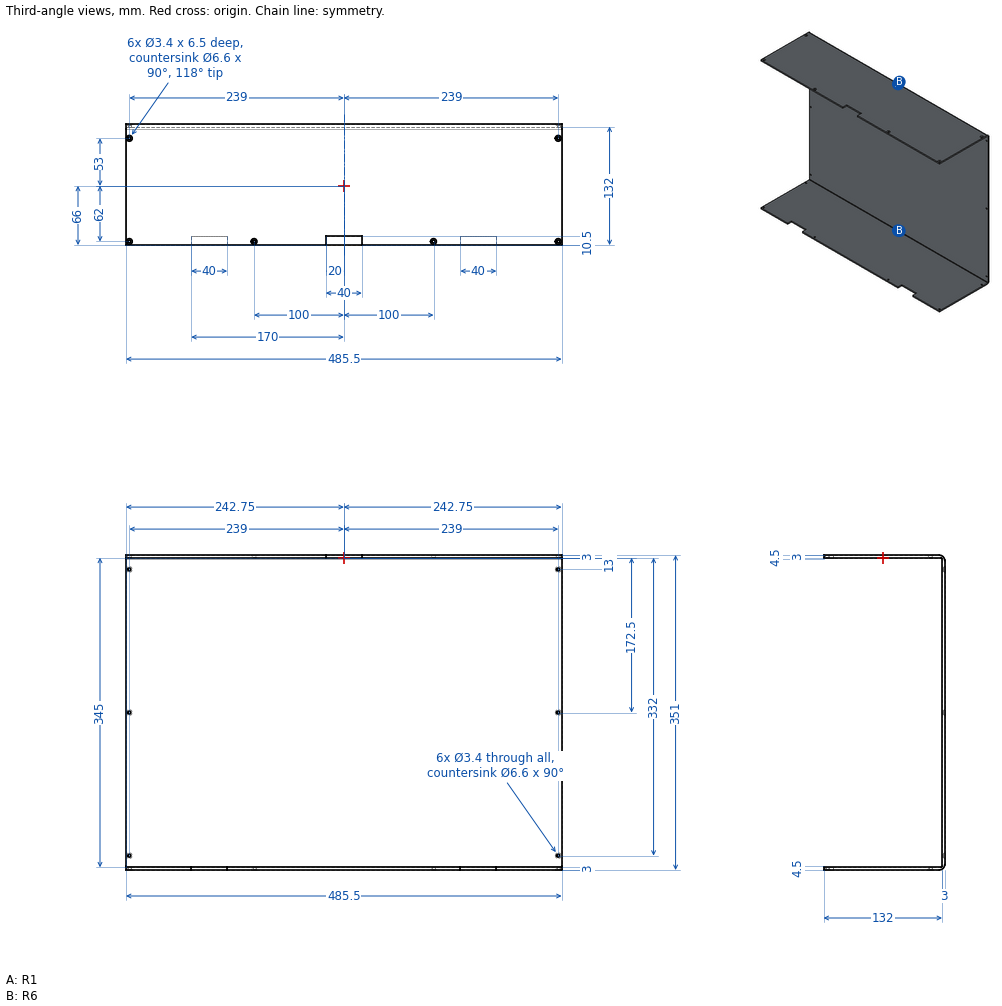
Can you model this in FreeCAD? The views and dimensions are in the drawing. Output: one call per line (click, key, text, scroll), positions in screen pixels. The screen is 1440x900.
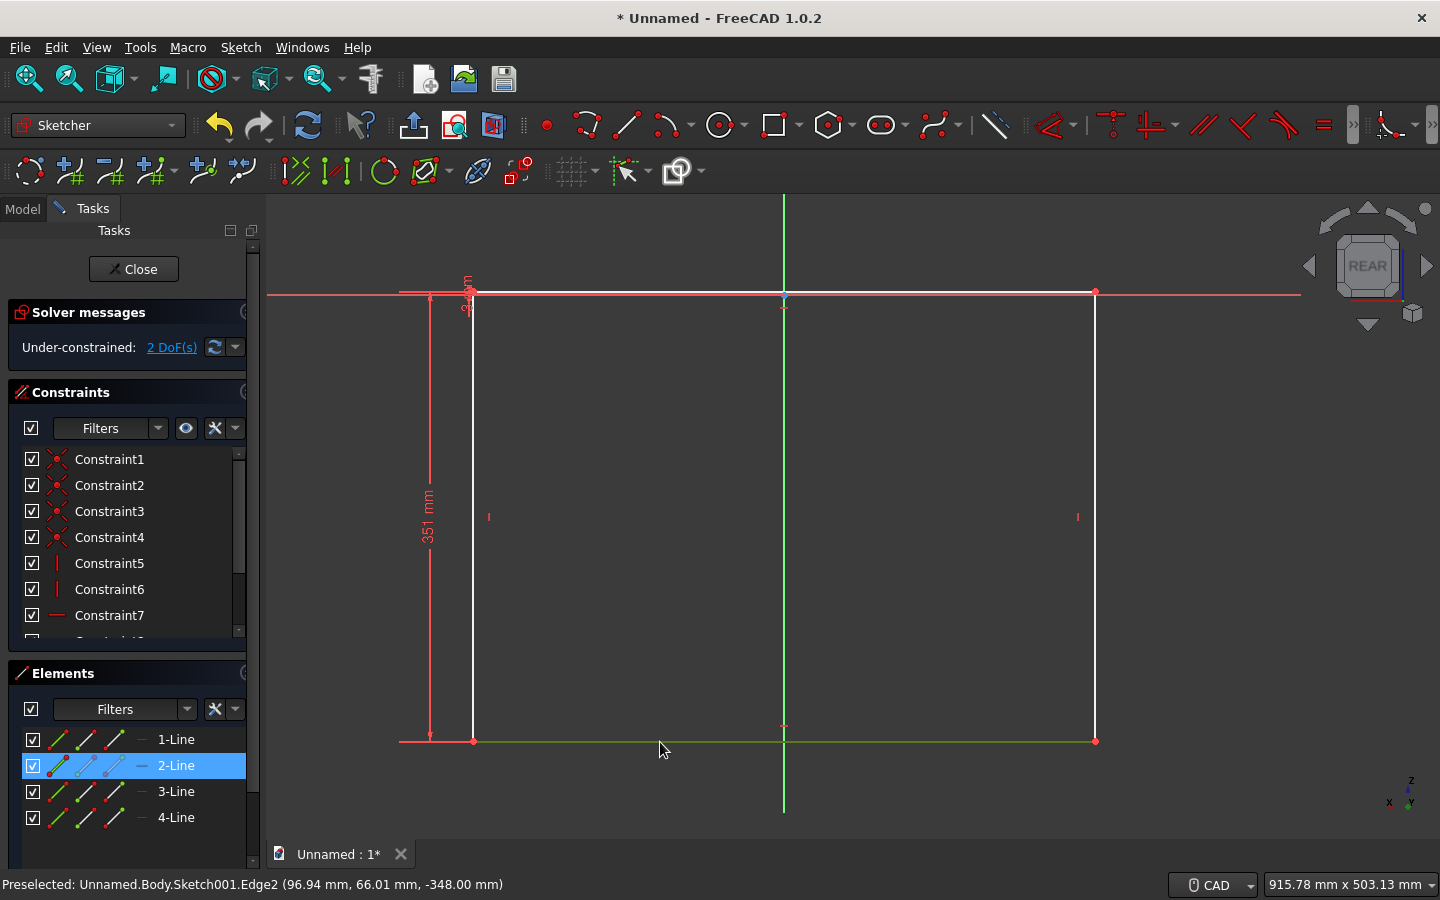
click(1076, 126)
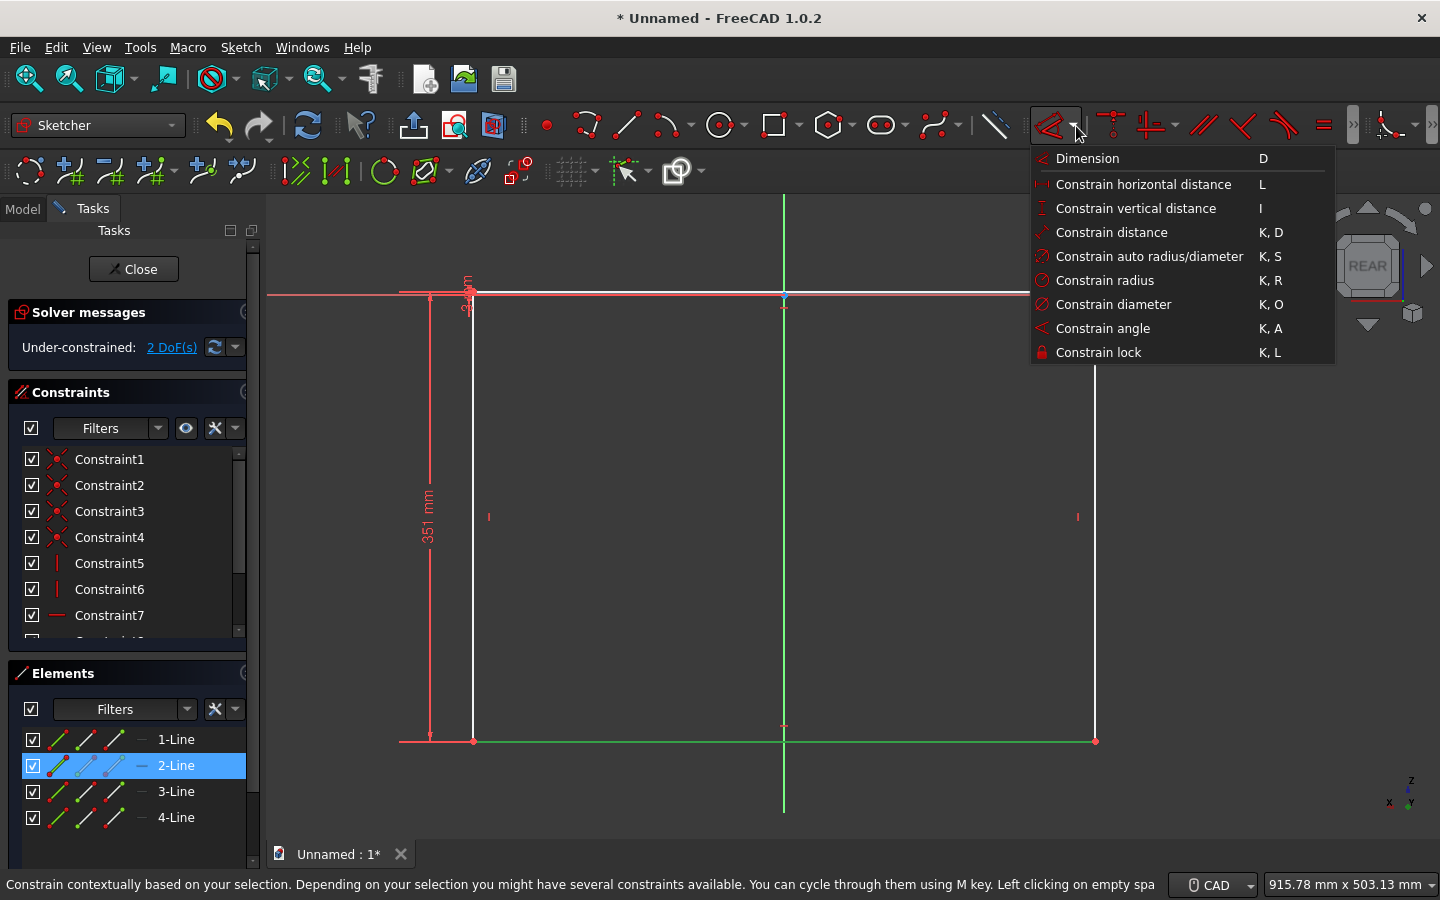
click(1183, 184)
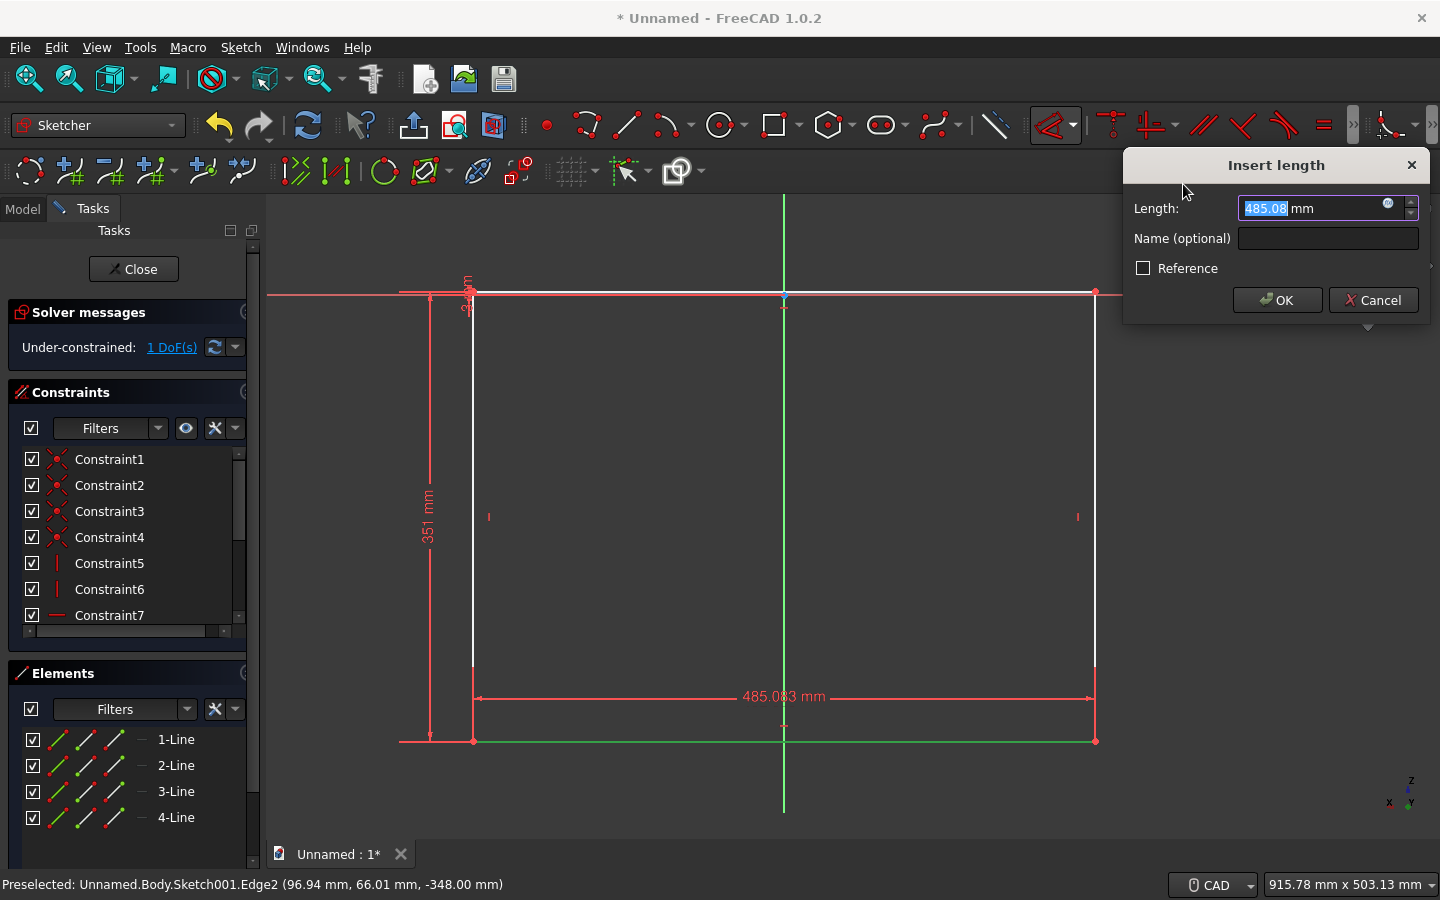
text(485.5)
key(Return)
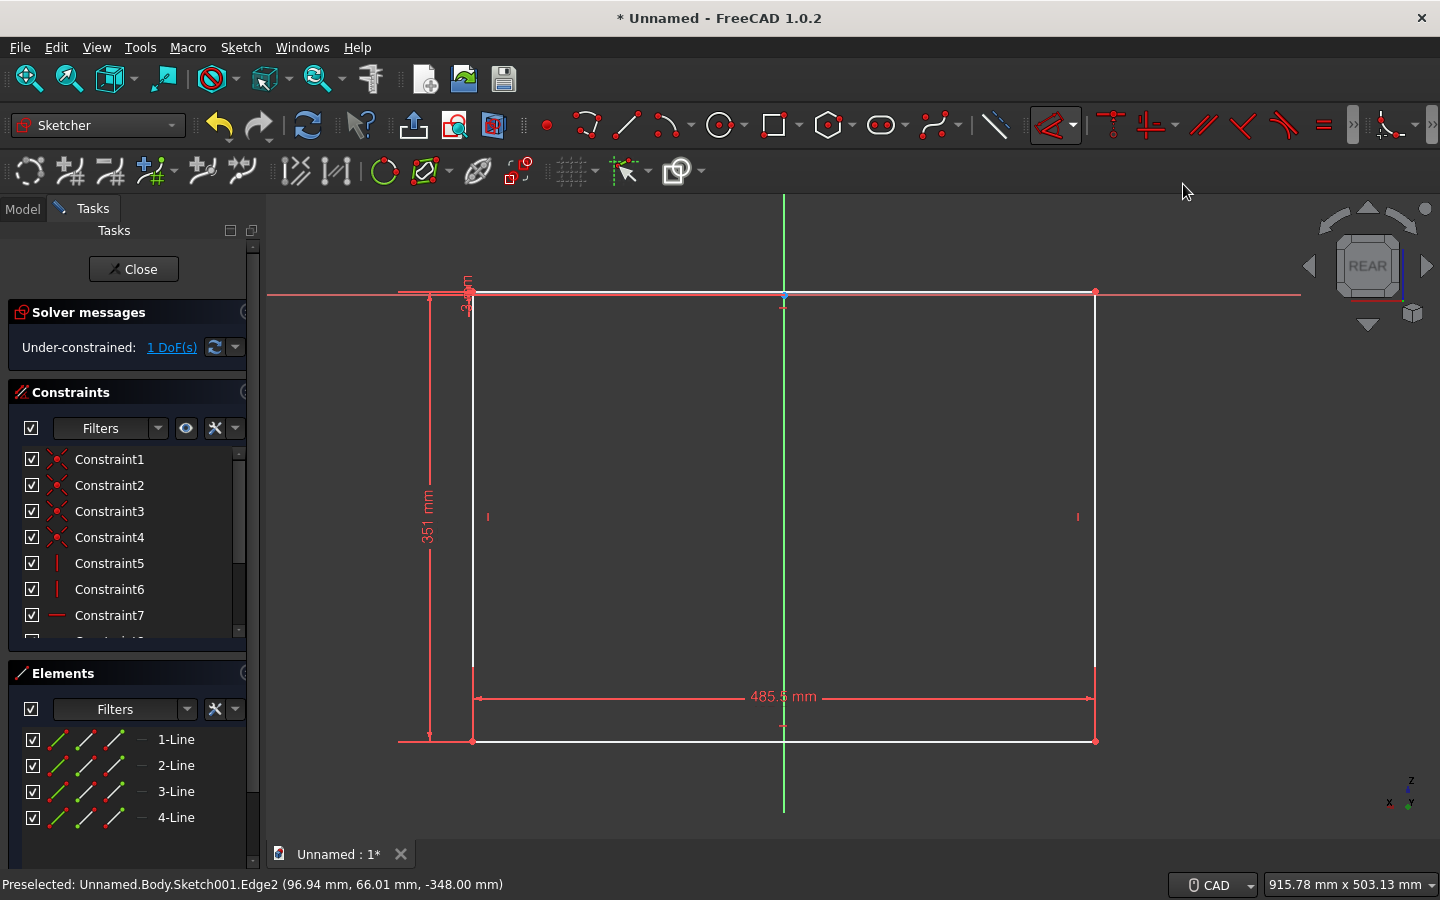
click(473, 292)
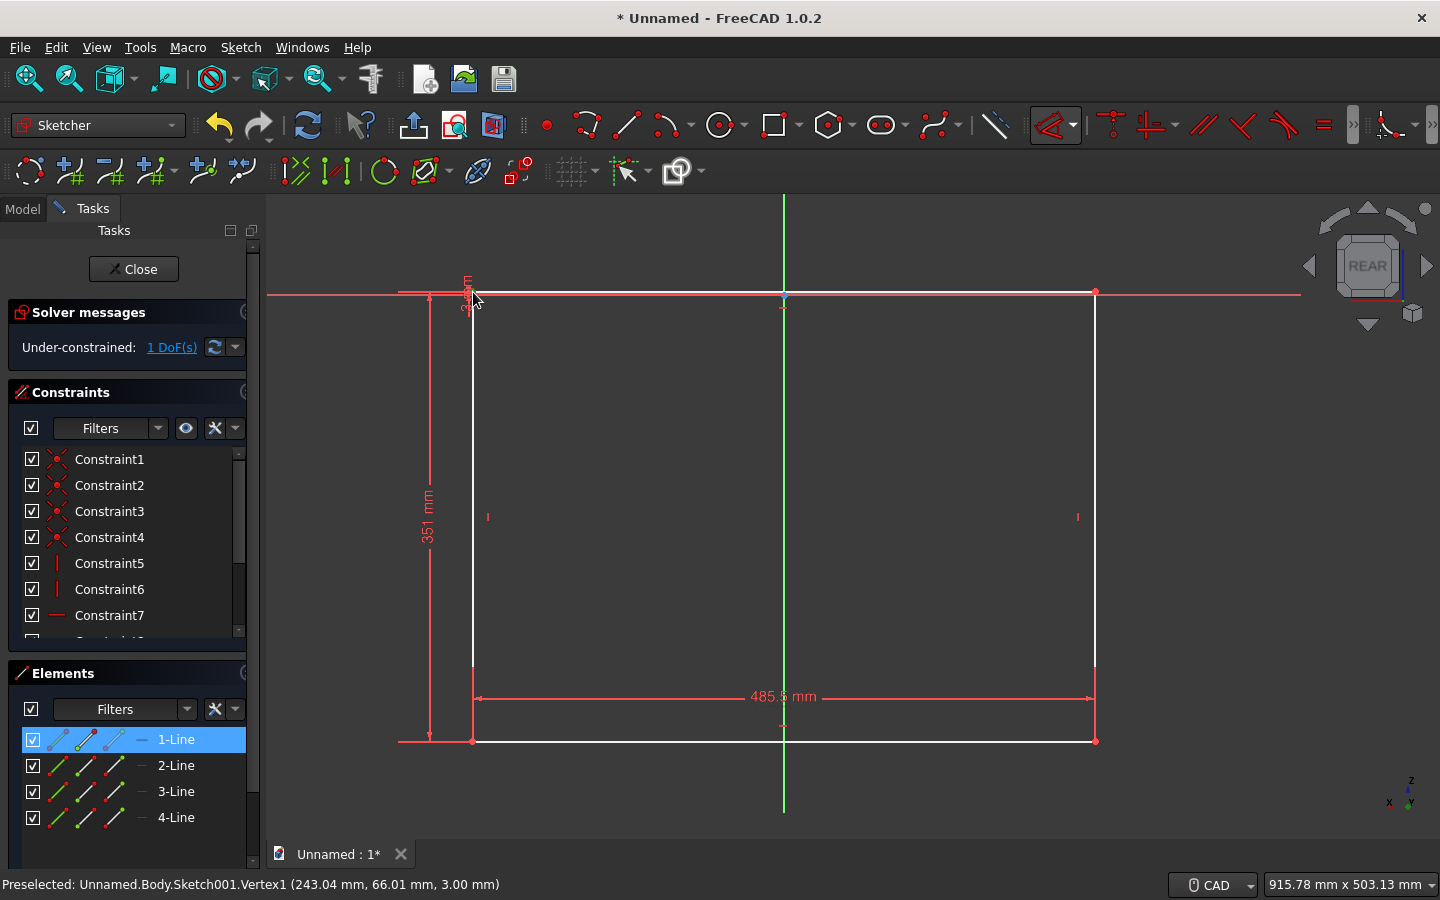
click(1076, 126)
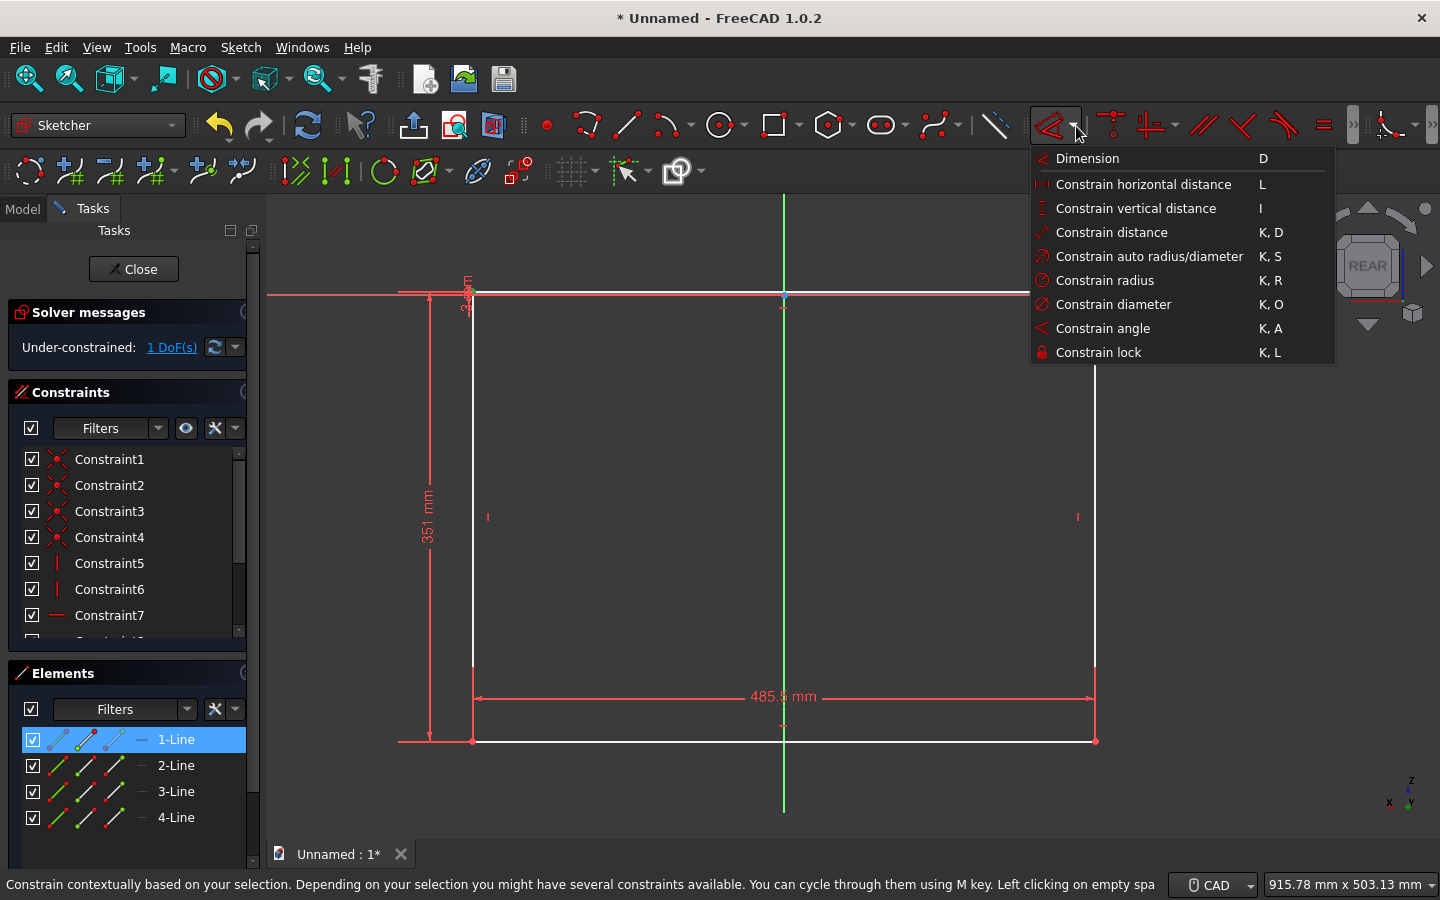
click(1183, 184)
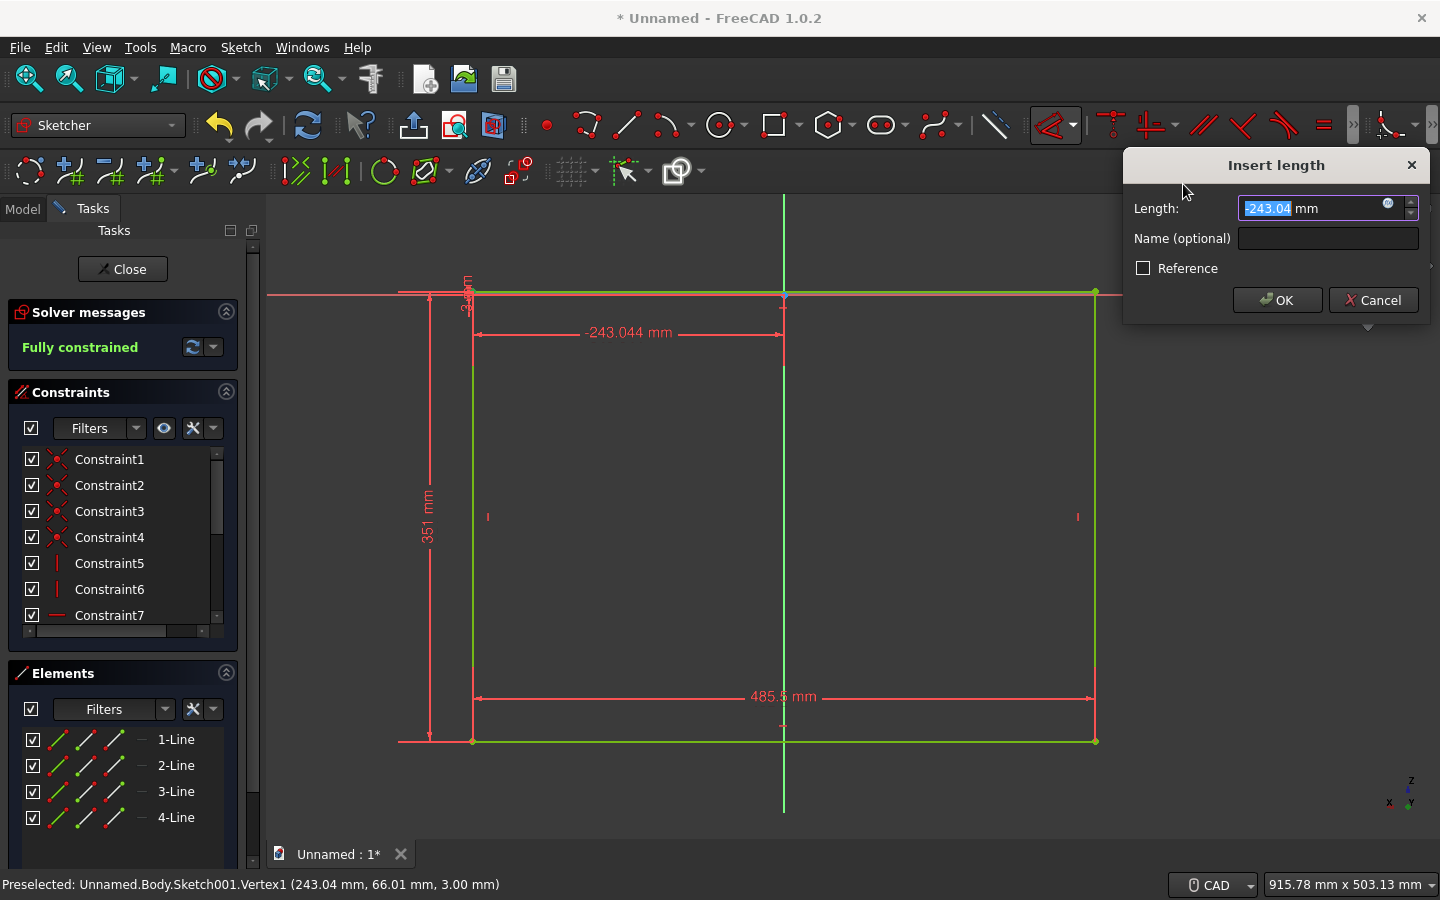
text(-242.75)
key(Return)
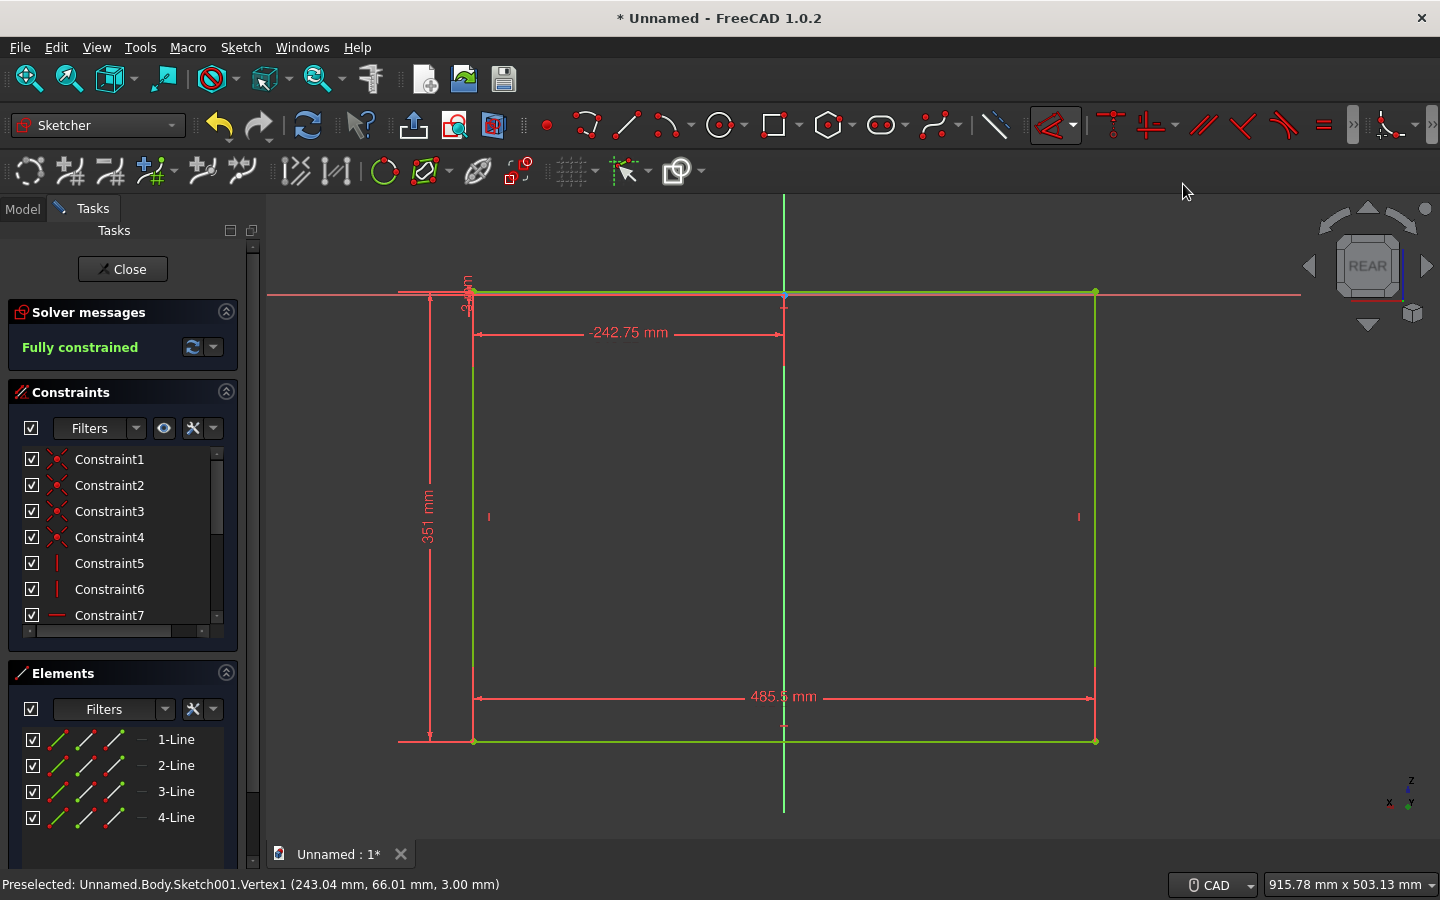
click(123, 269)